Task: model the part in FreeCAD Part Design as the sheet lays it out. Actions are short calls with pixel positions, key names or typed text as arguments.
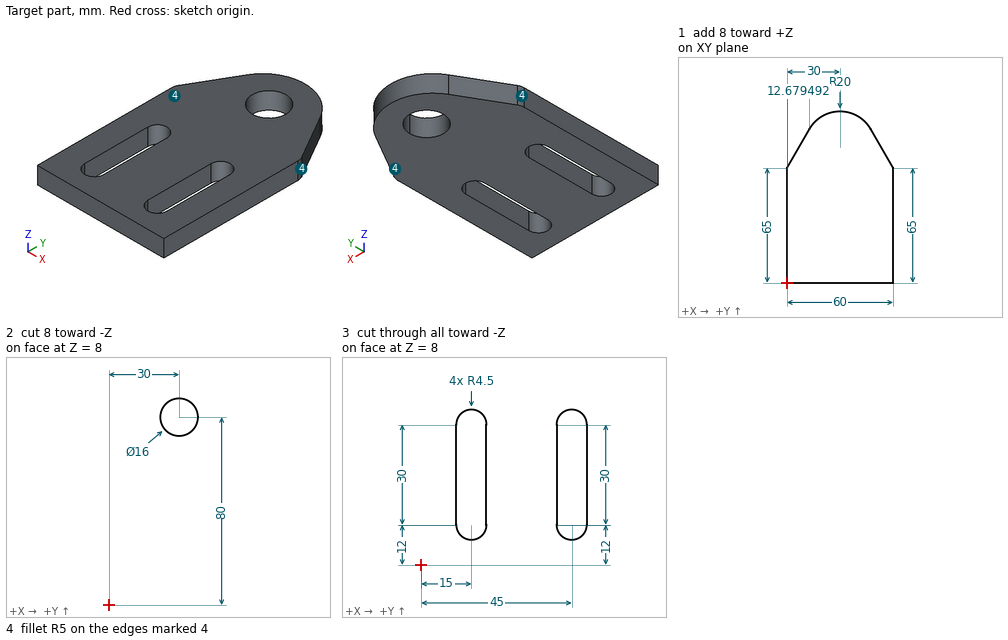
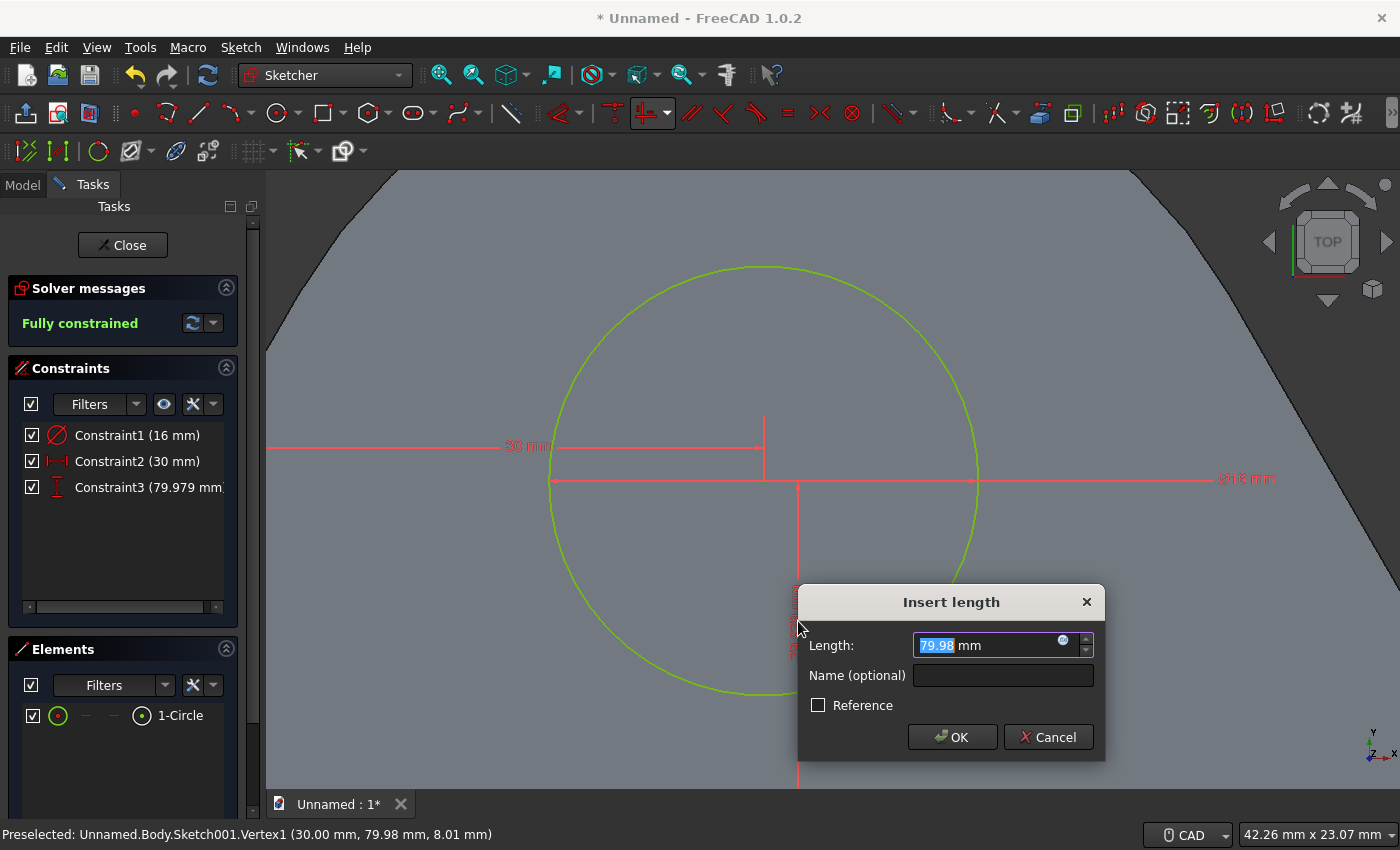
text(80)
key(Return)
key(Escape)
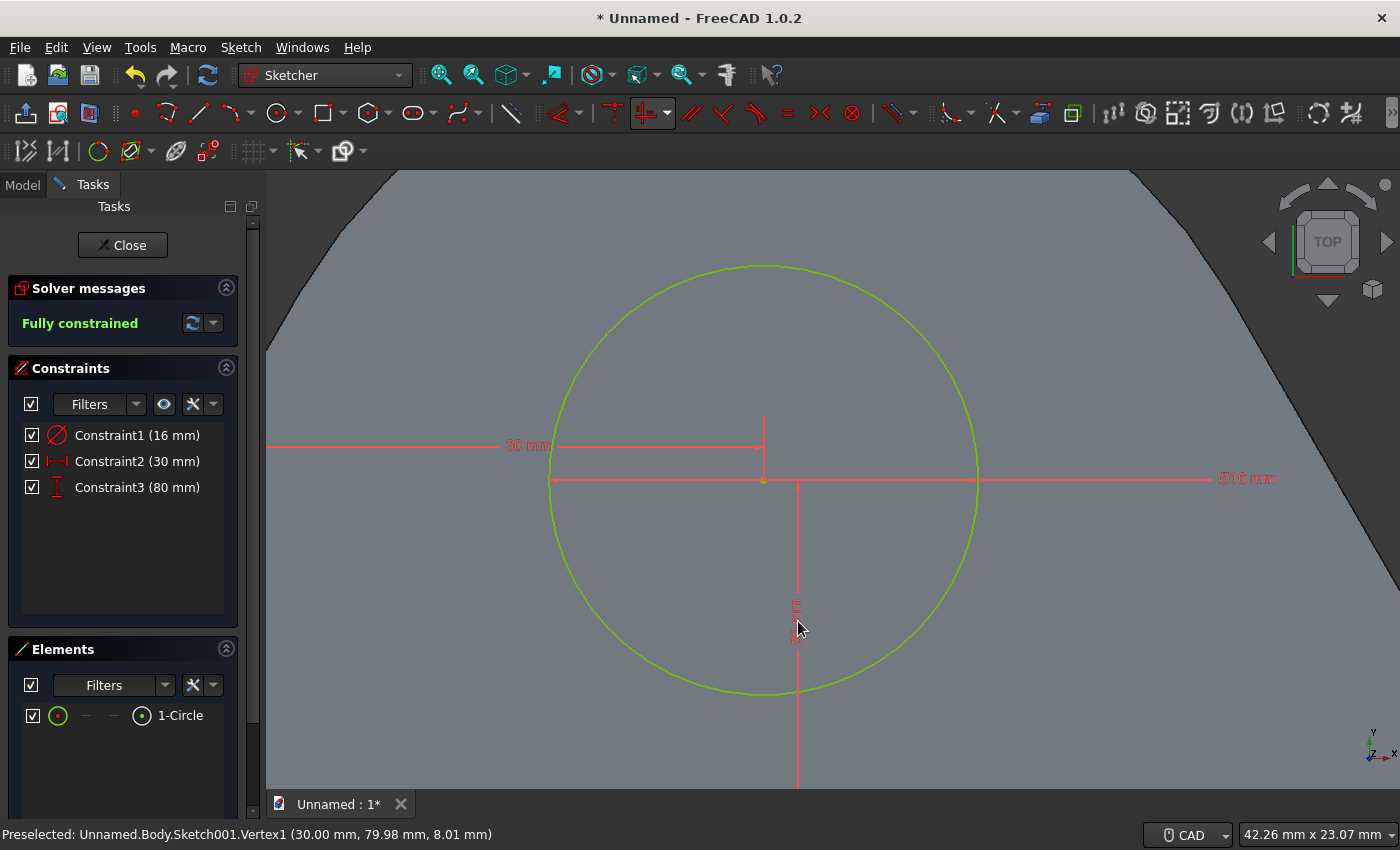
click(123, 245)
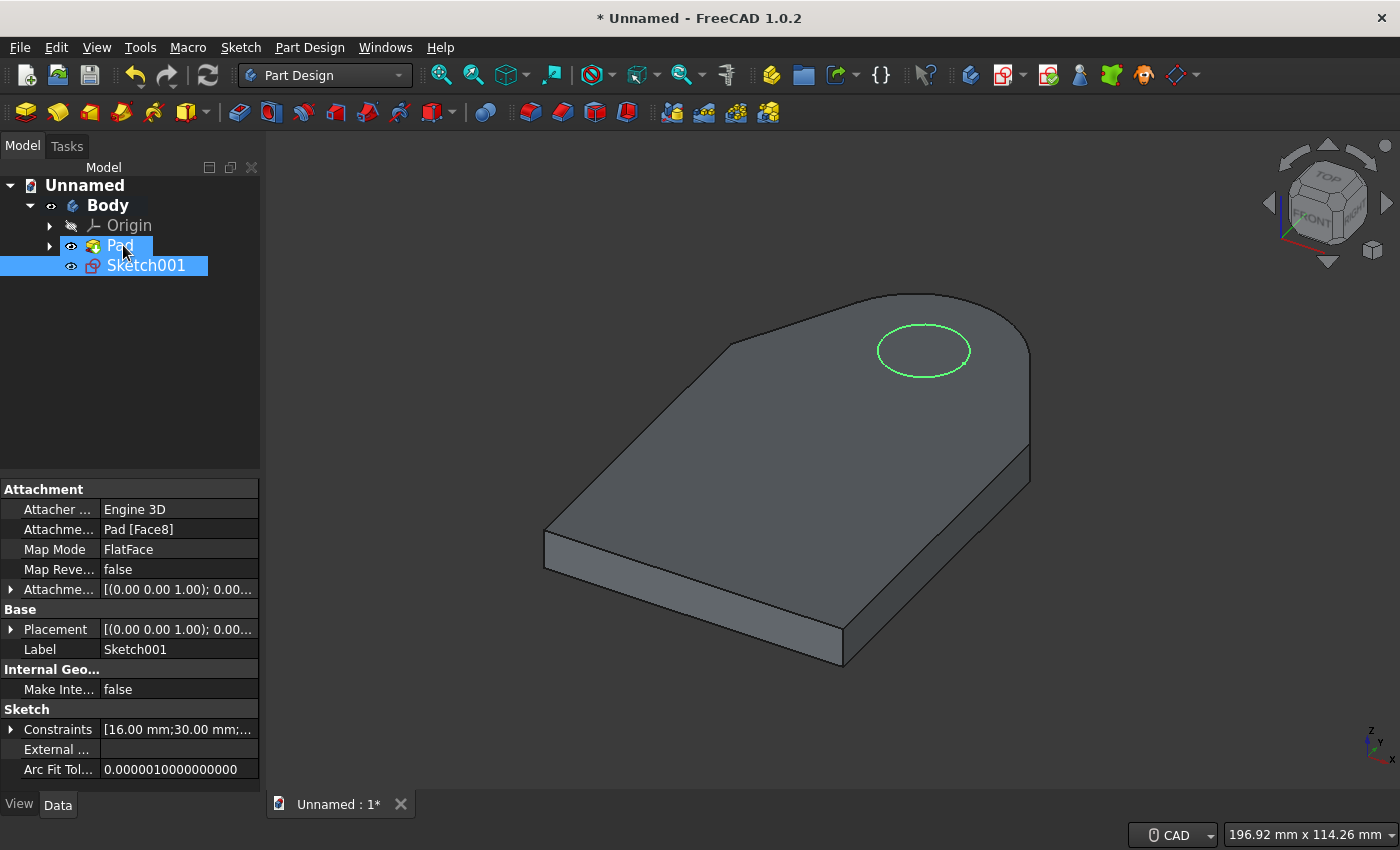
click(240, 112)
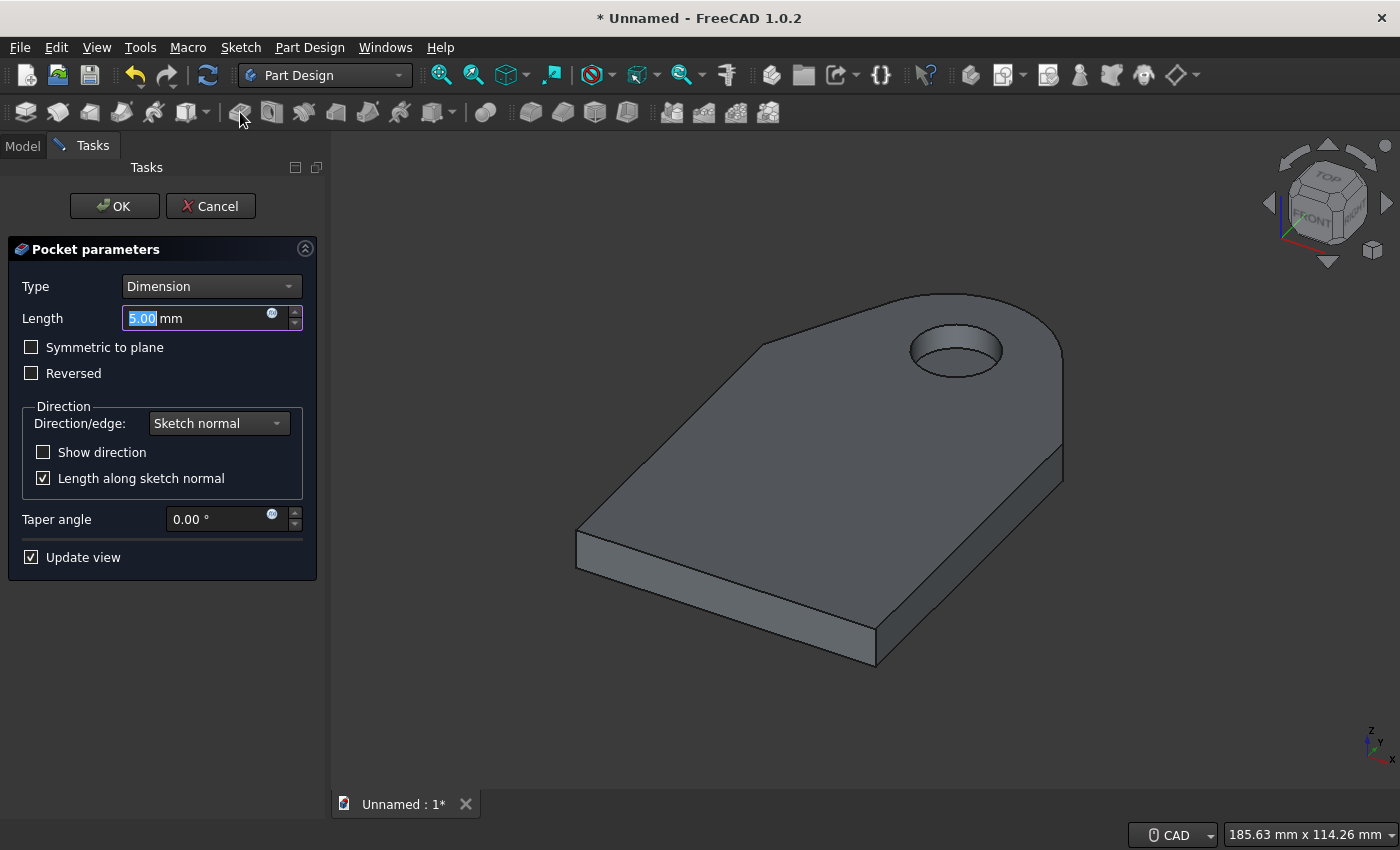
text(8)
key(Tab)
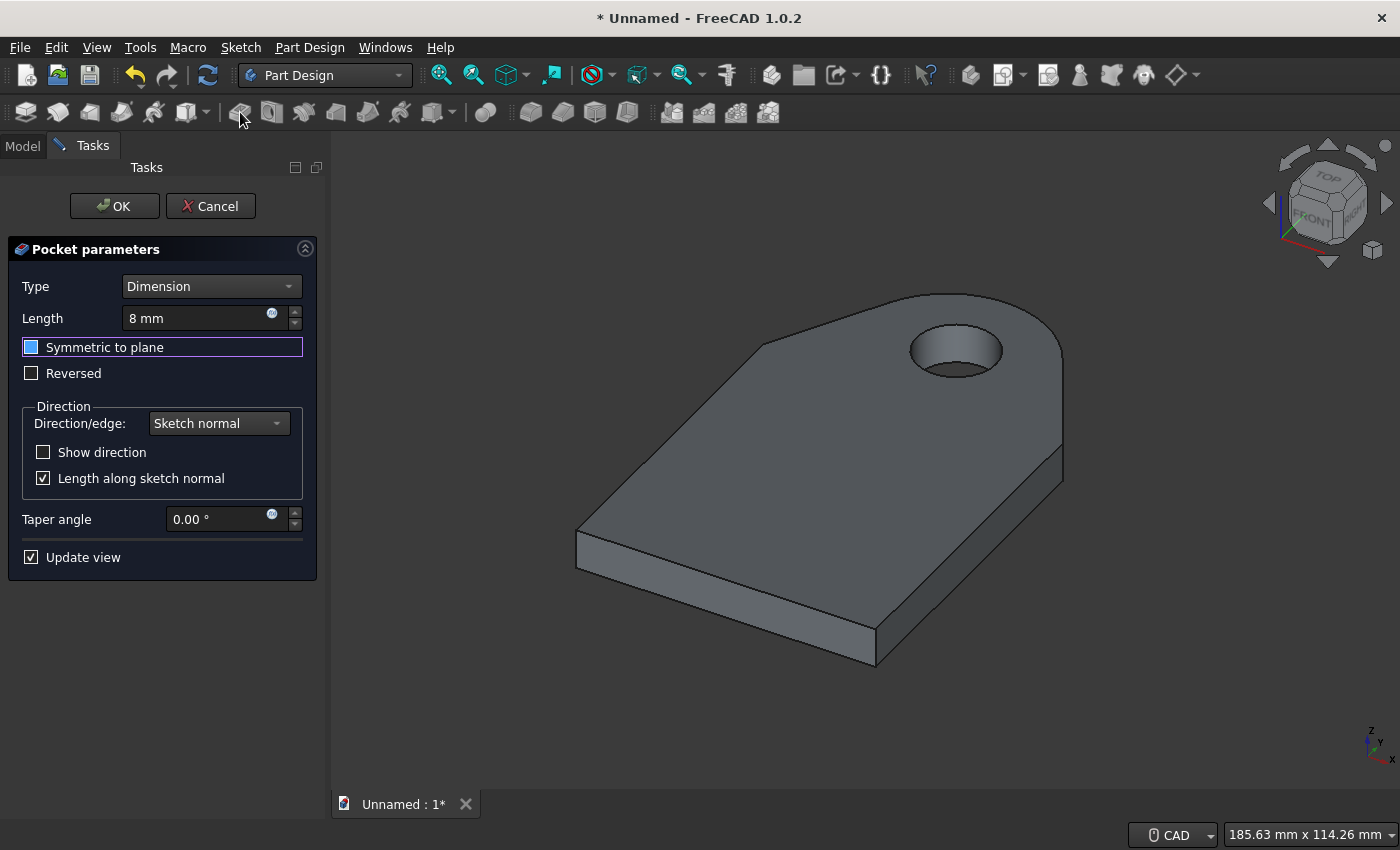
click(115, 206)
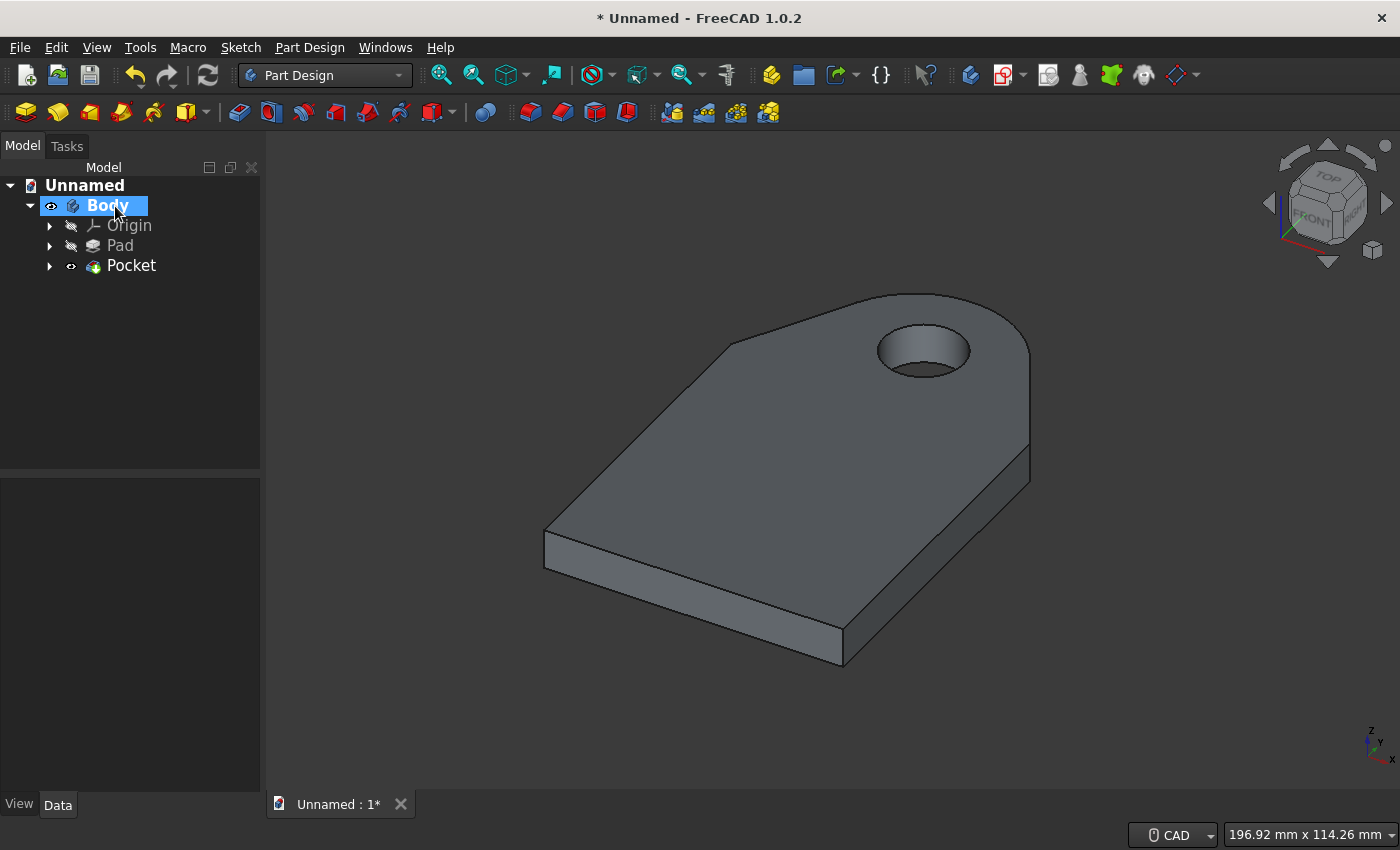
click(793, 480)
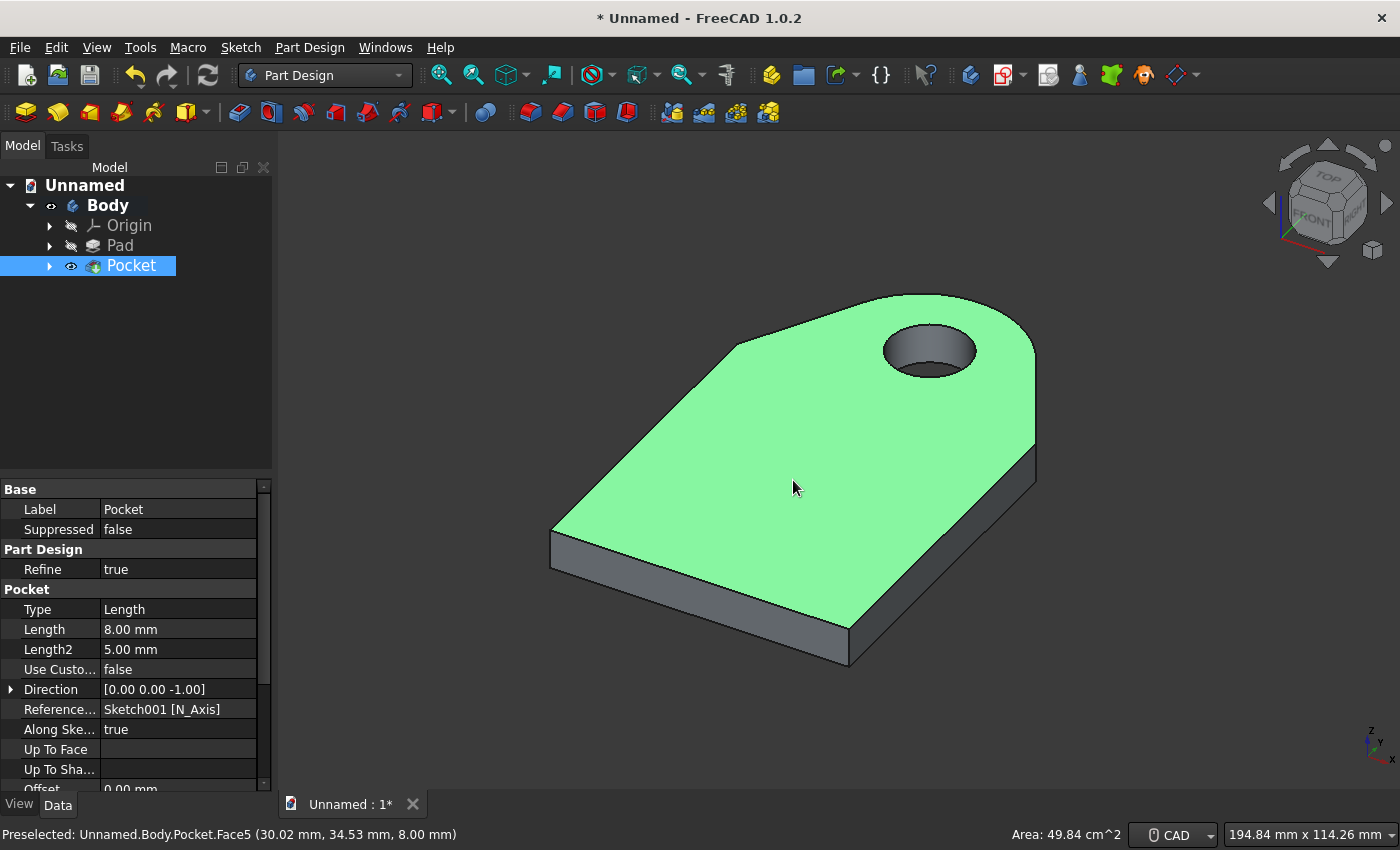
click(1004, 76)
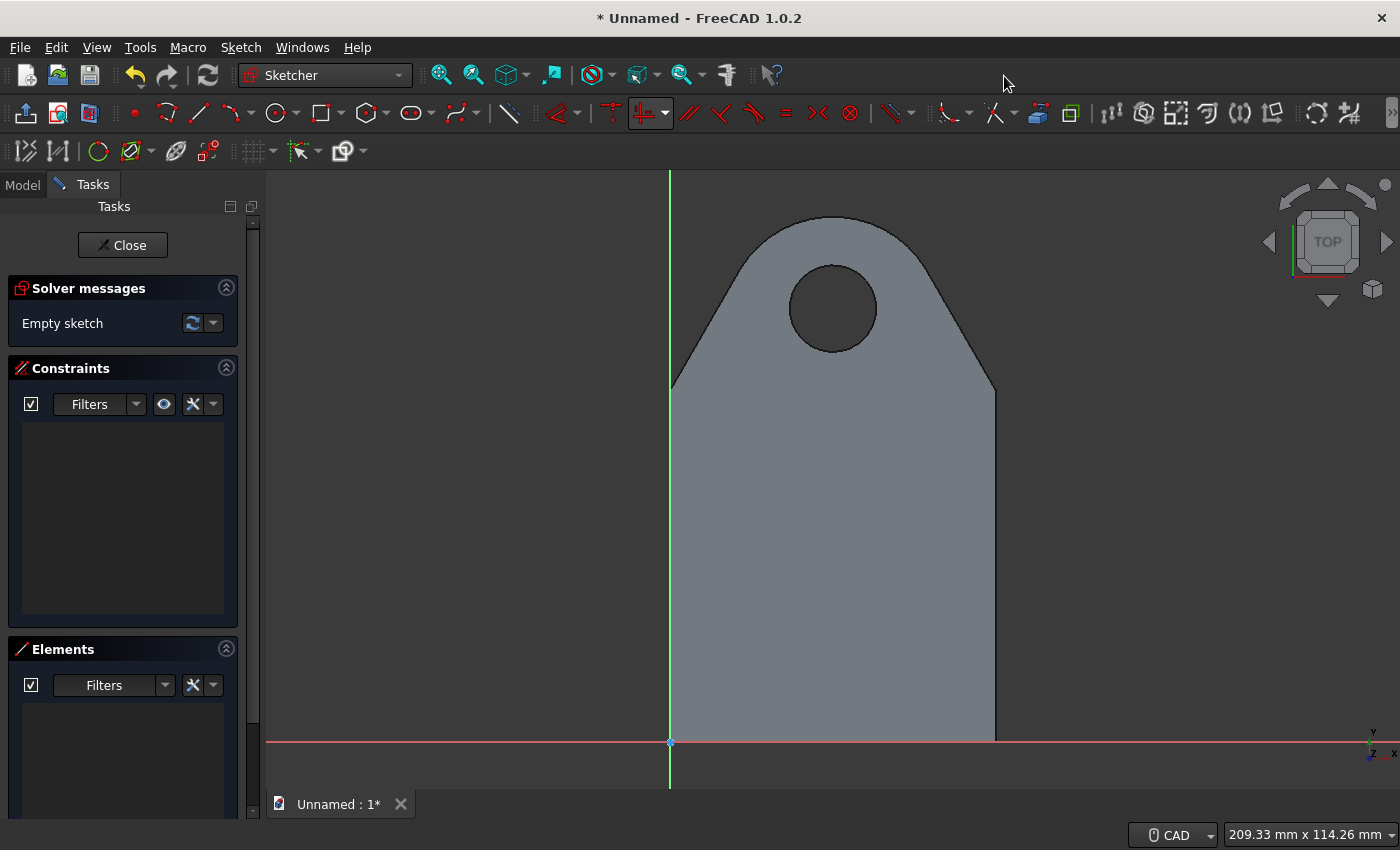
scroll(886, 761, up, 2)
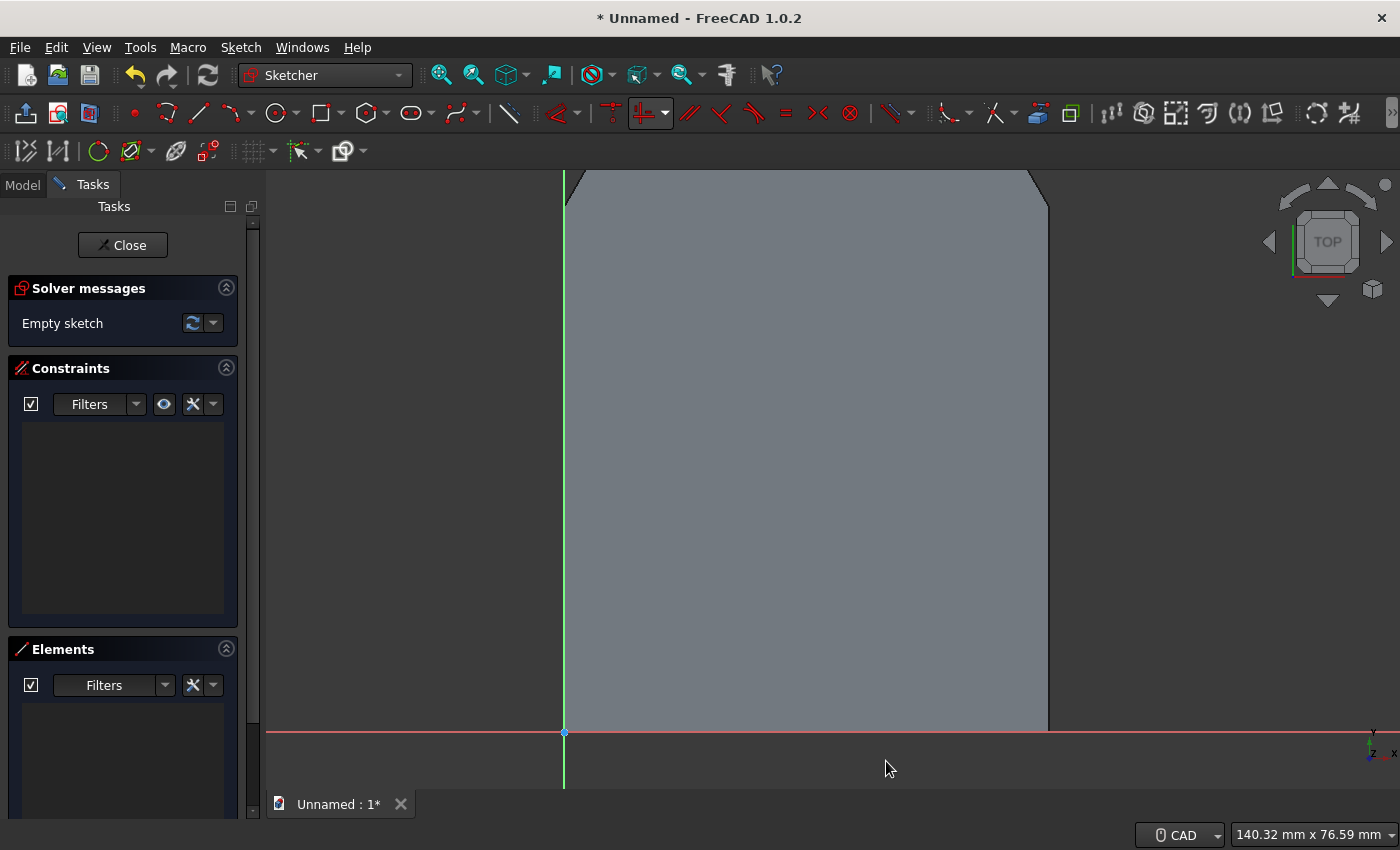
key(g)
key(s)